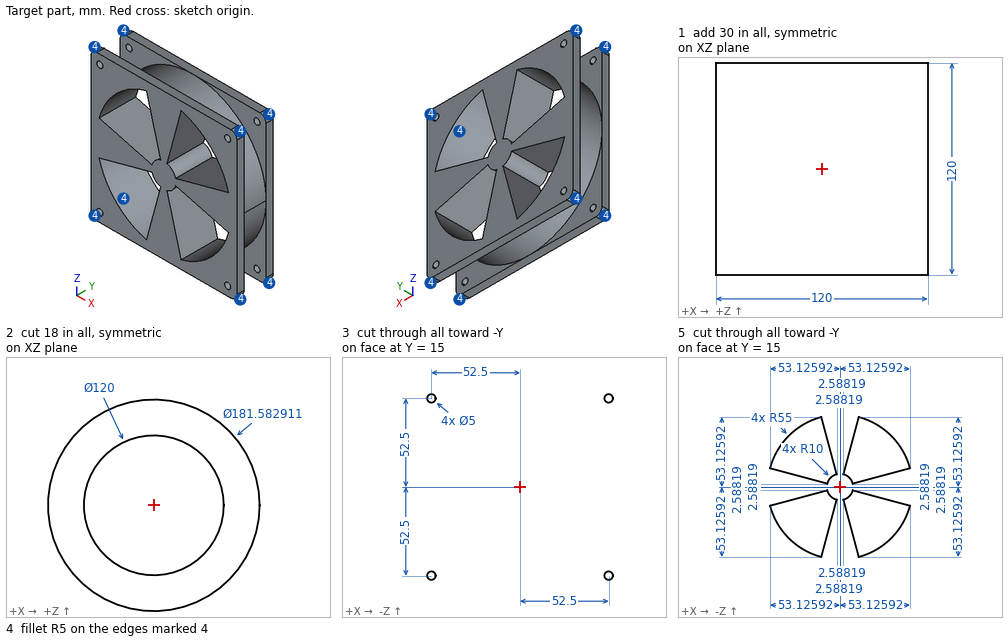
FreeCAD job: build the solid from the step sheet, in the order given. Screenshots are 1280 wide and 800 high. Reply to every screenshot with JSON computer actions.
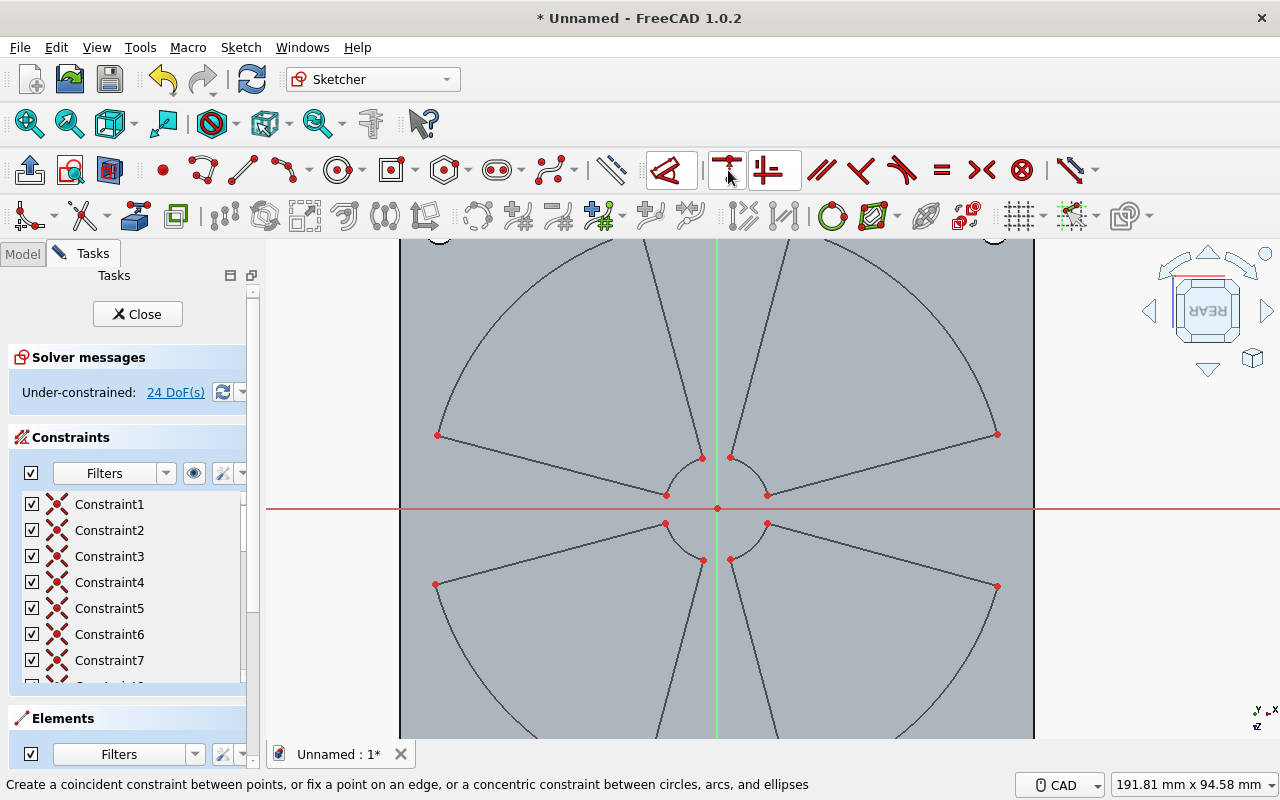
{"action": "left_click", "coordinate": [688, 465]}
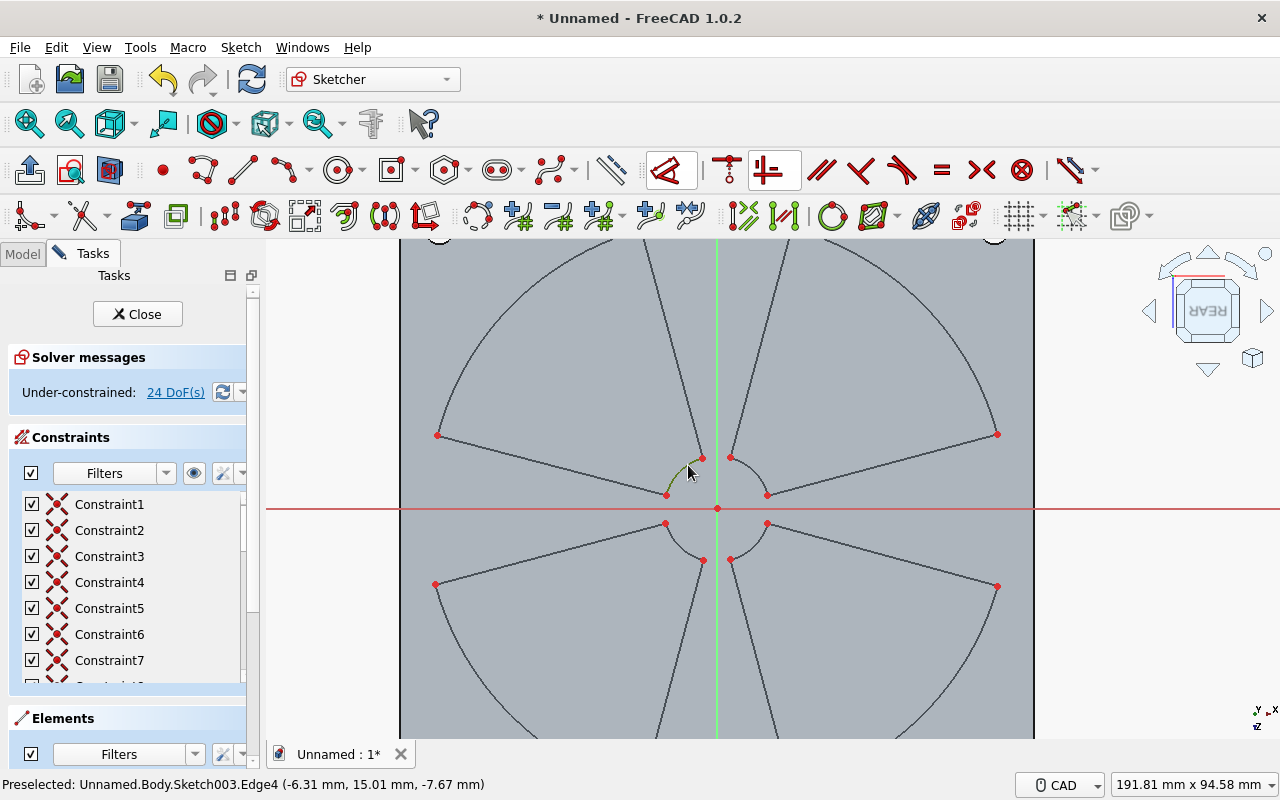
{"action": "left_click", "coordinate": [761, 480]}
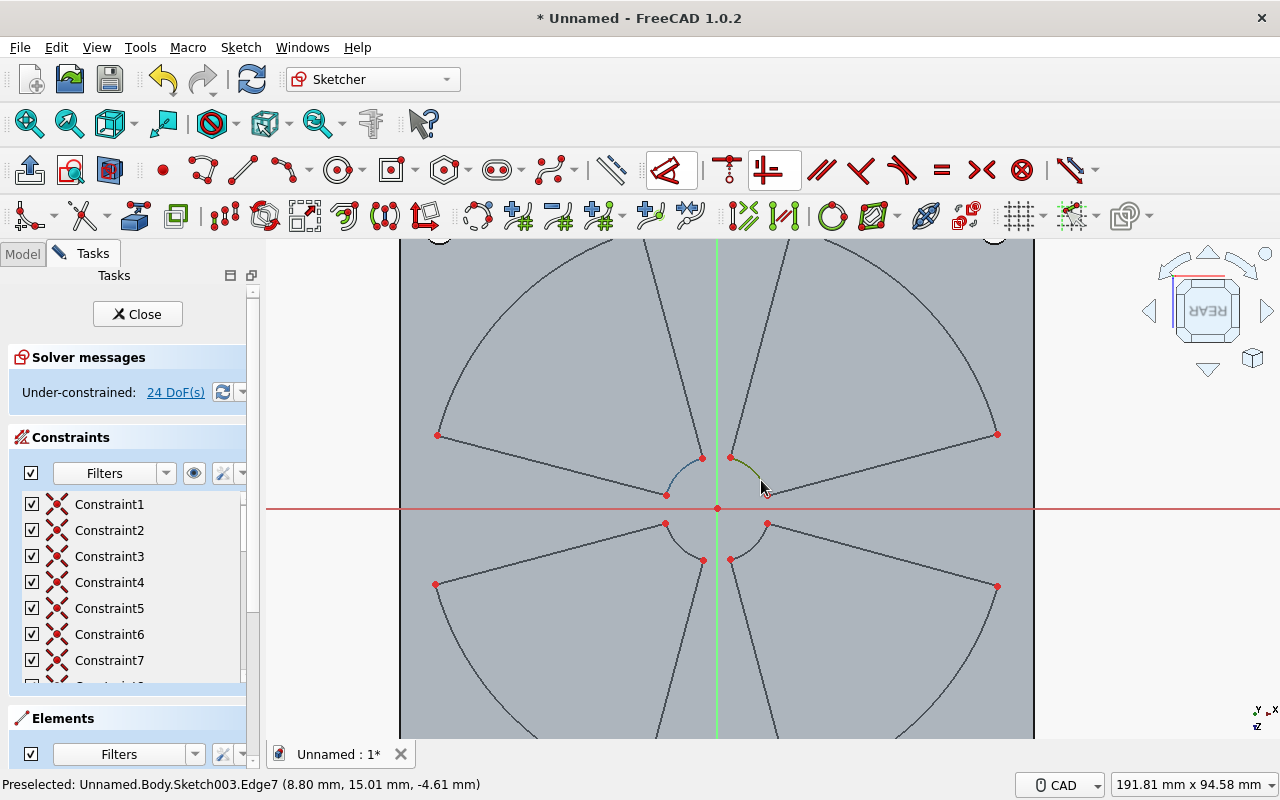
{"action": "left_click", "coordinate": [745, 553]}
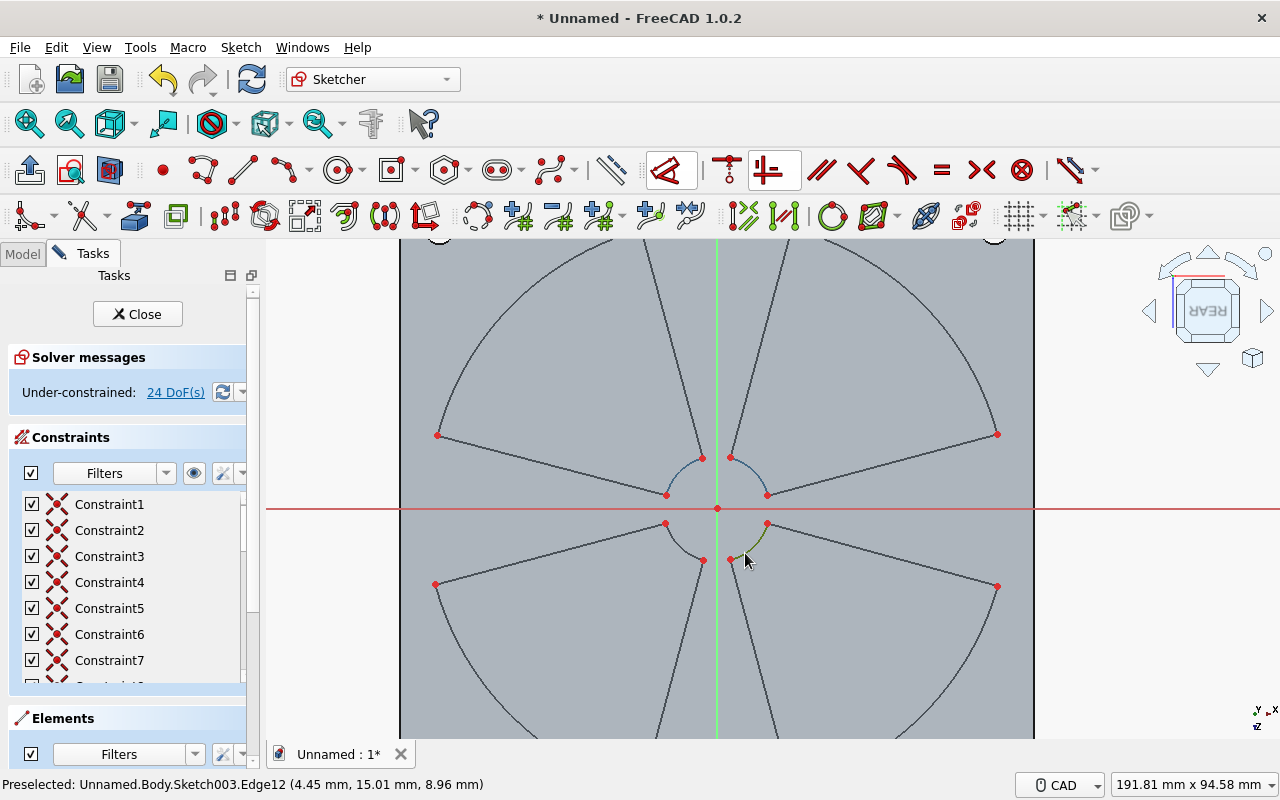
{"action": "left_click", "coordinate": [673, 538]}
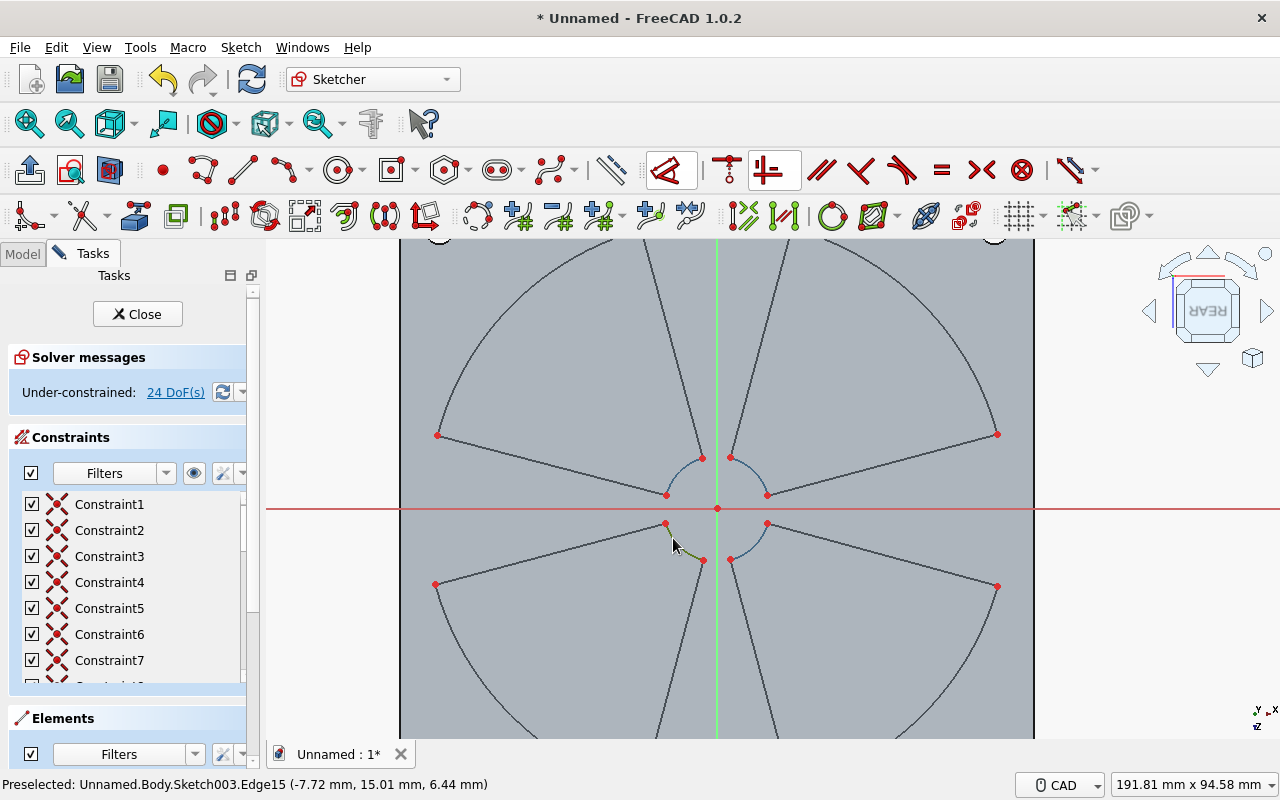
{"action": "left_click", "coordinate": [942, 170]}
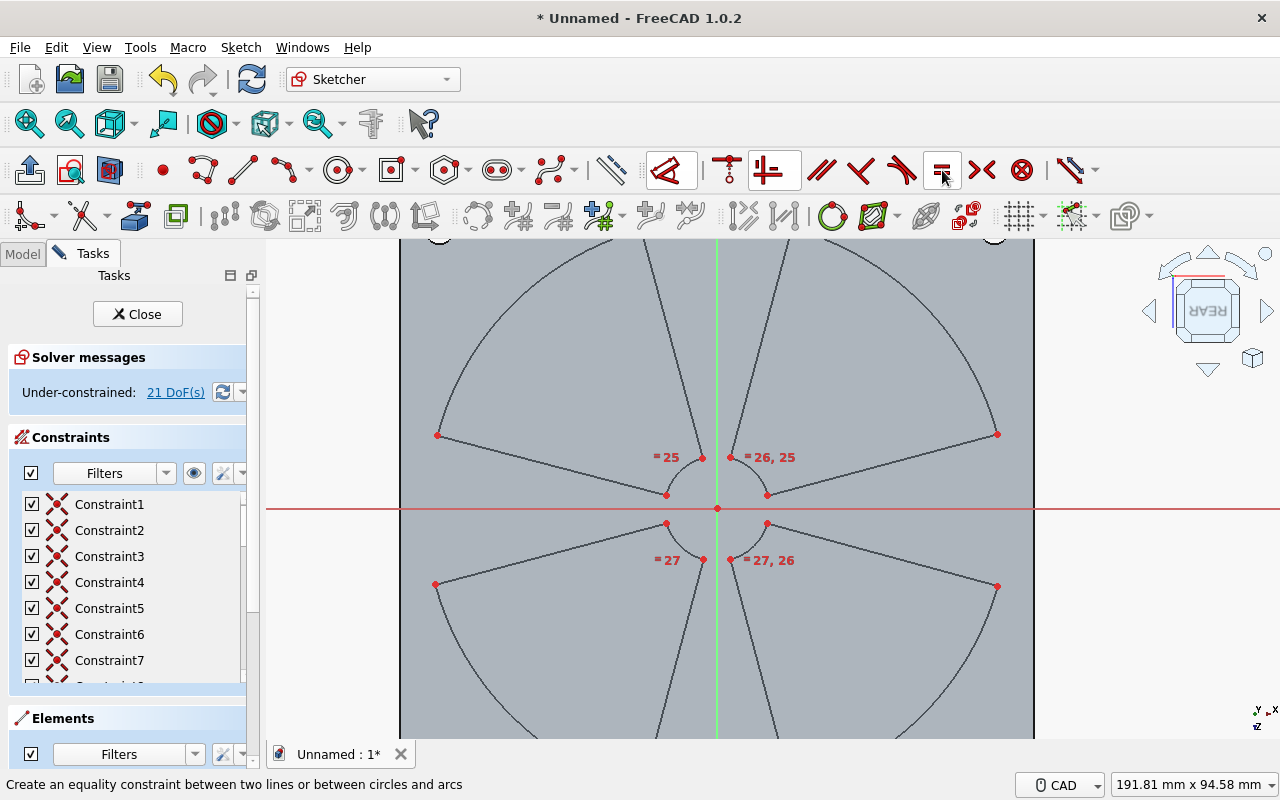
{"action": "left_click", "coordinate": [559, 267]}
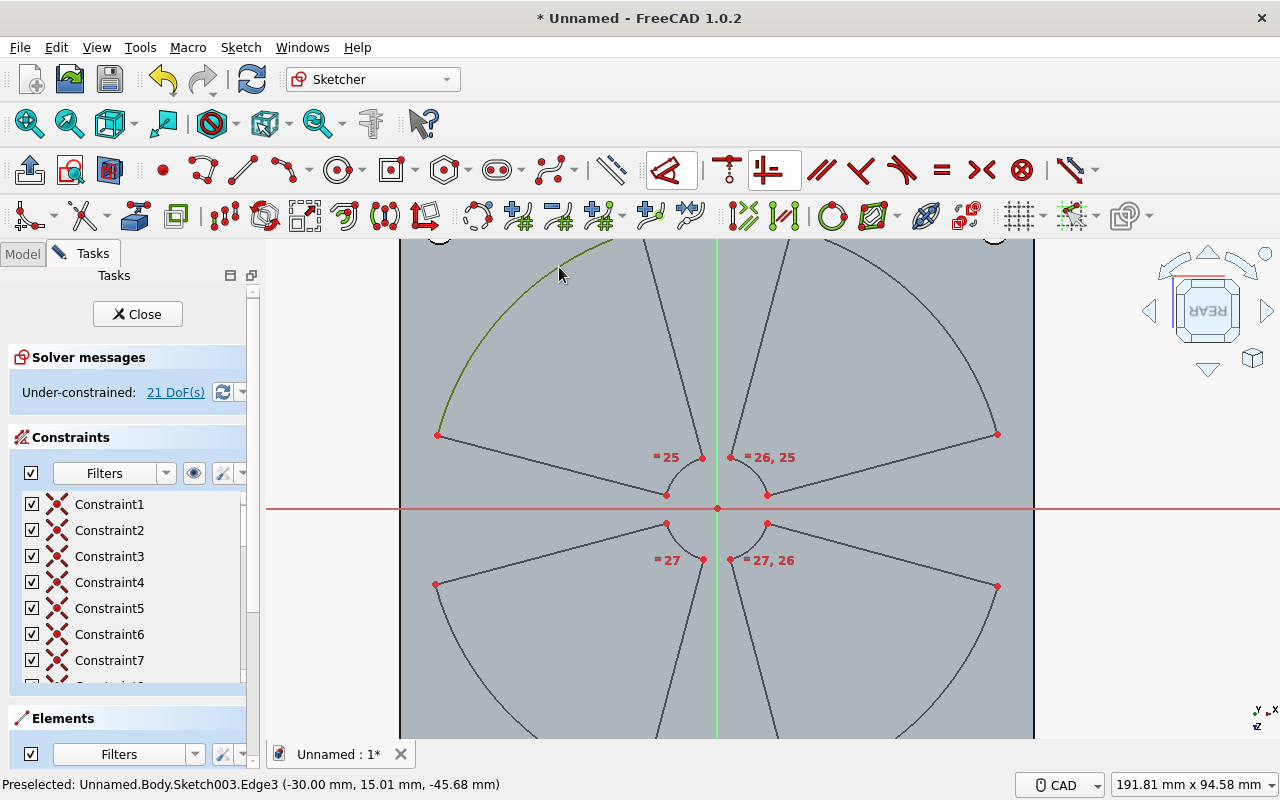
{"action": "left_click", "coordinate": [961, 351]}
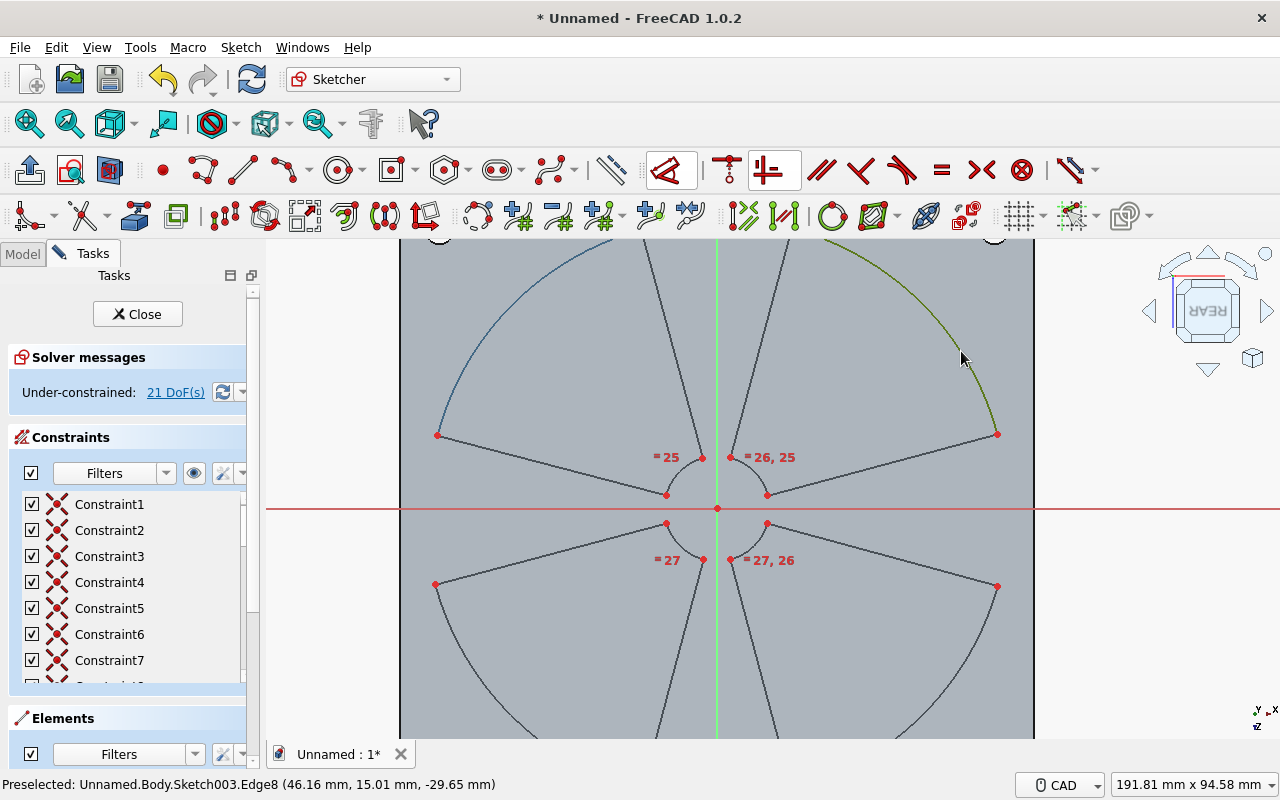
{"action": "left_click", "coordinate": [960, 669]}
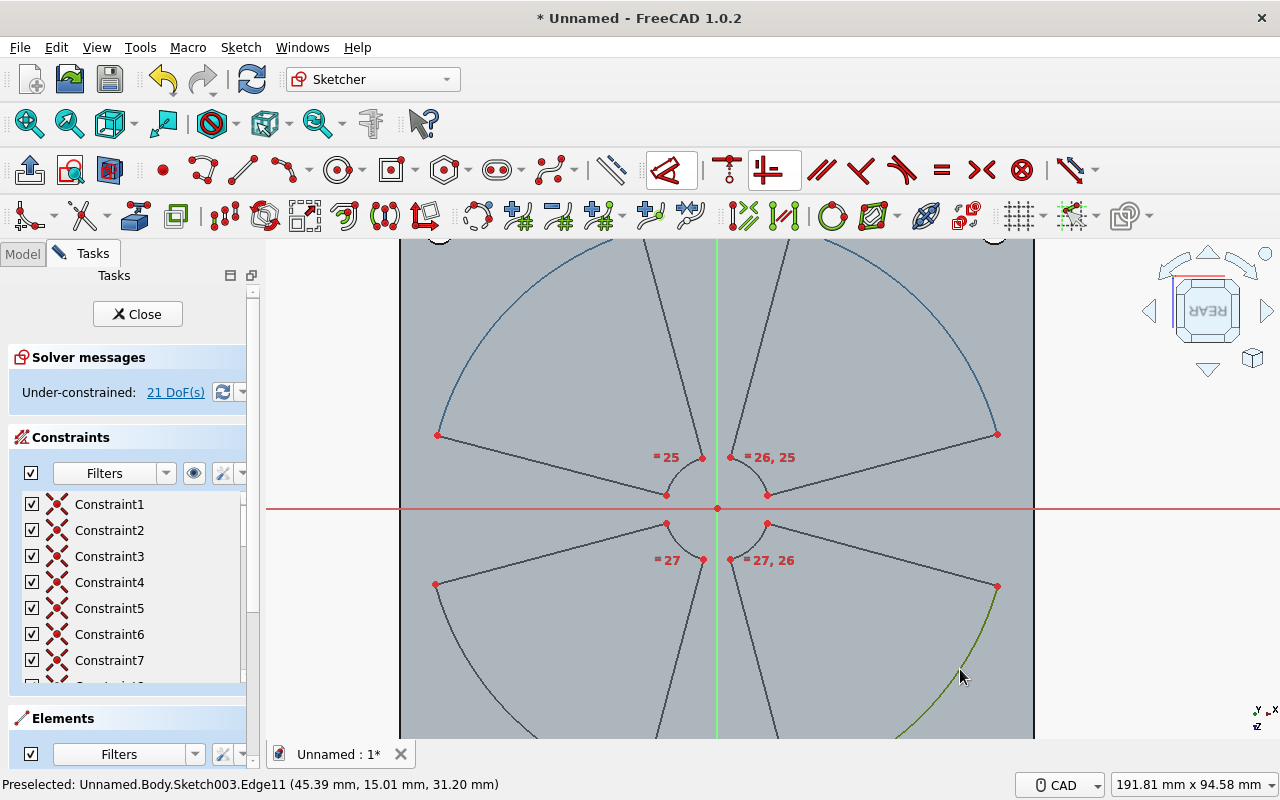
{"action": "left_click", "coordinate": [473, 668]}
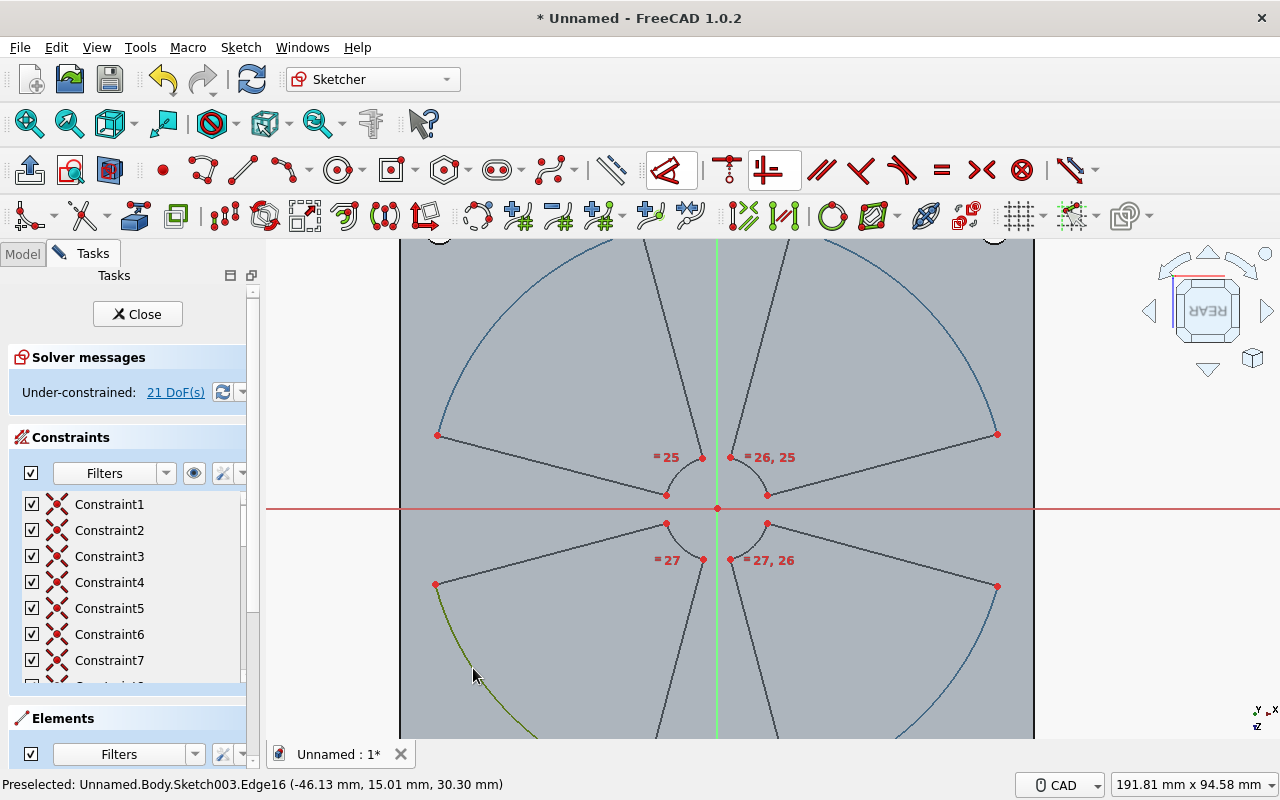
{"action": "left_click", "coordinate": [942, 170]}